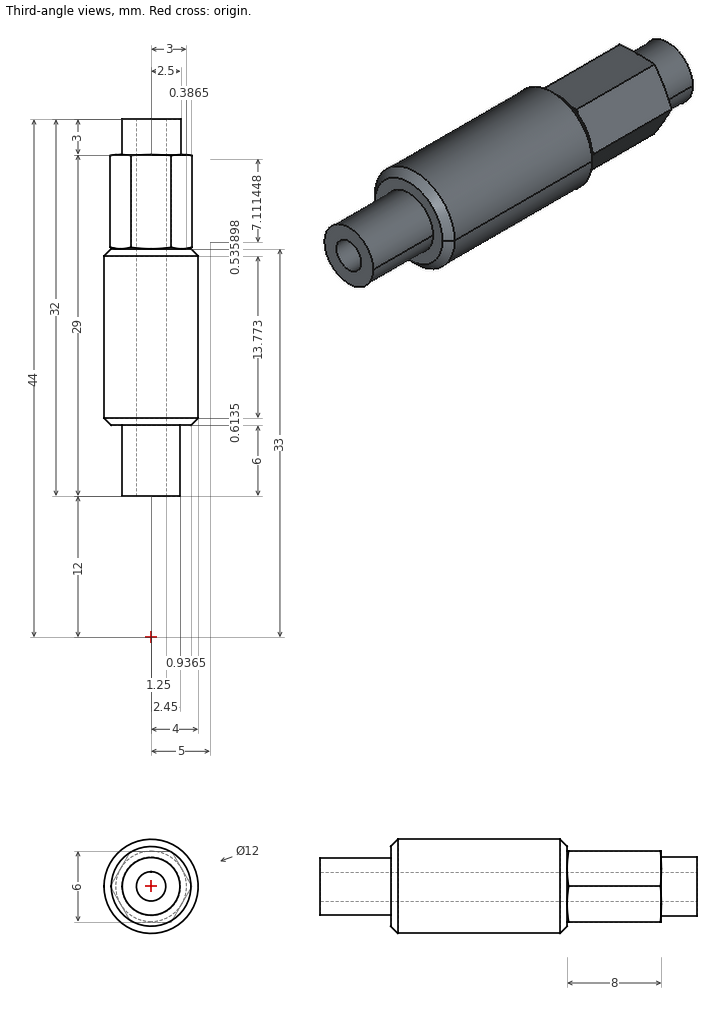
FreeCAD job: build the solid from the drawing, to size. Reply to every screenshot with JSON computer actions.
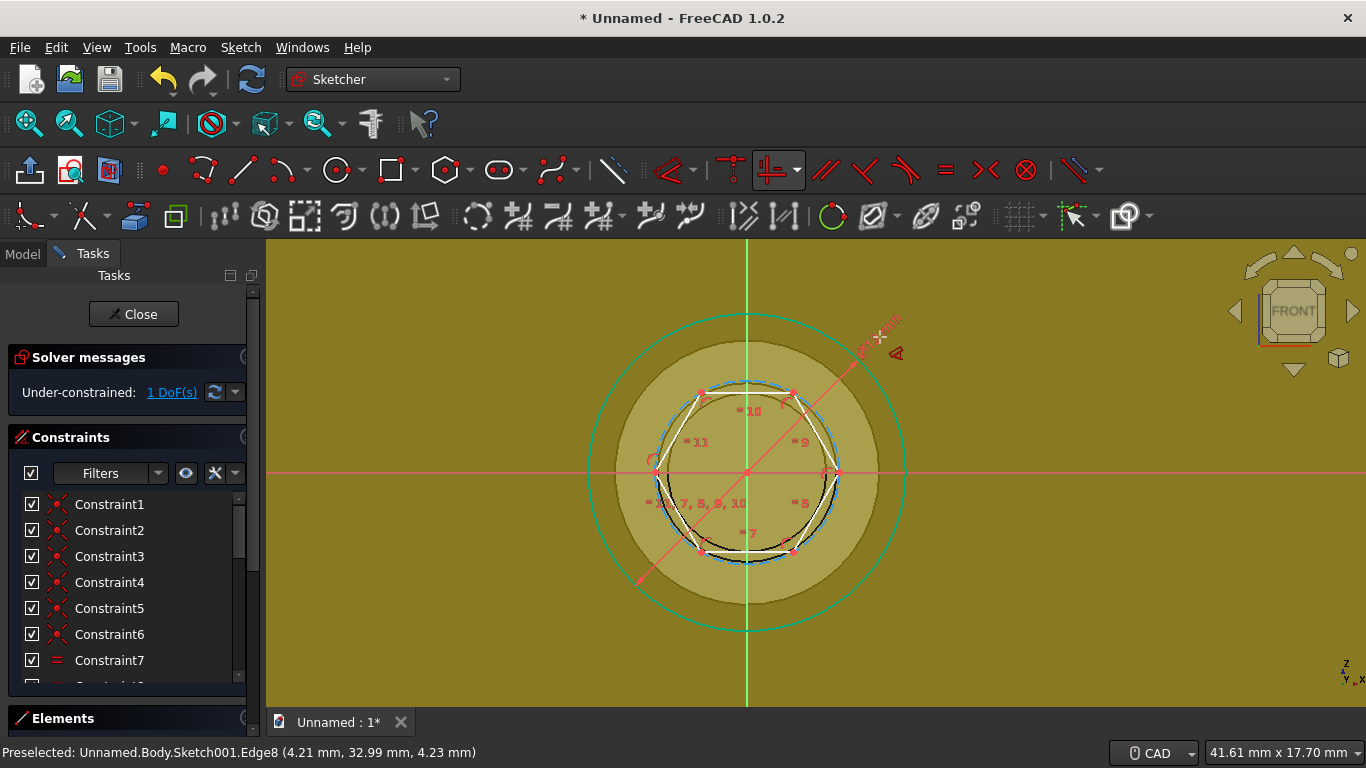
{"action": "left_click", "coordinate": [701, 552]}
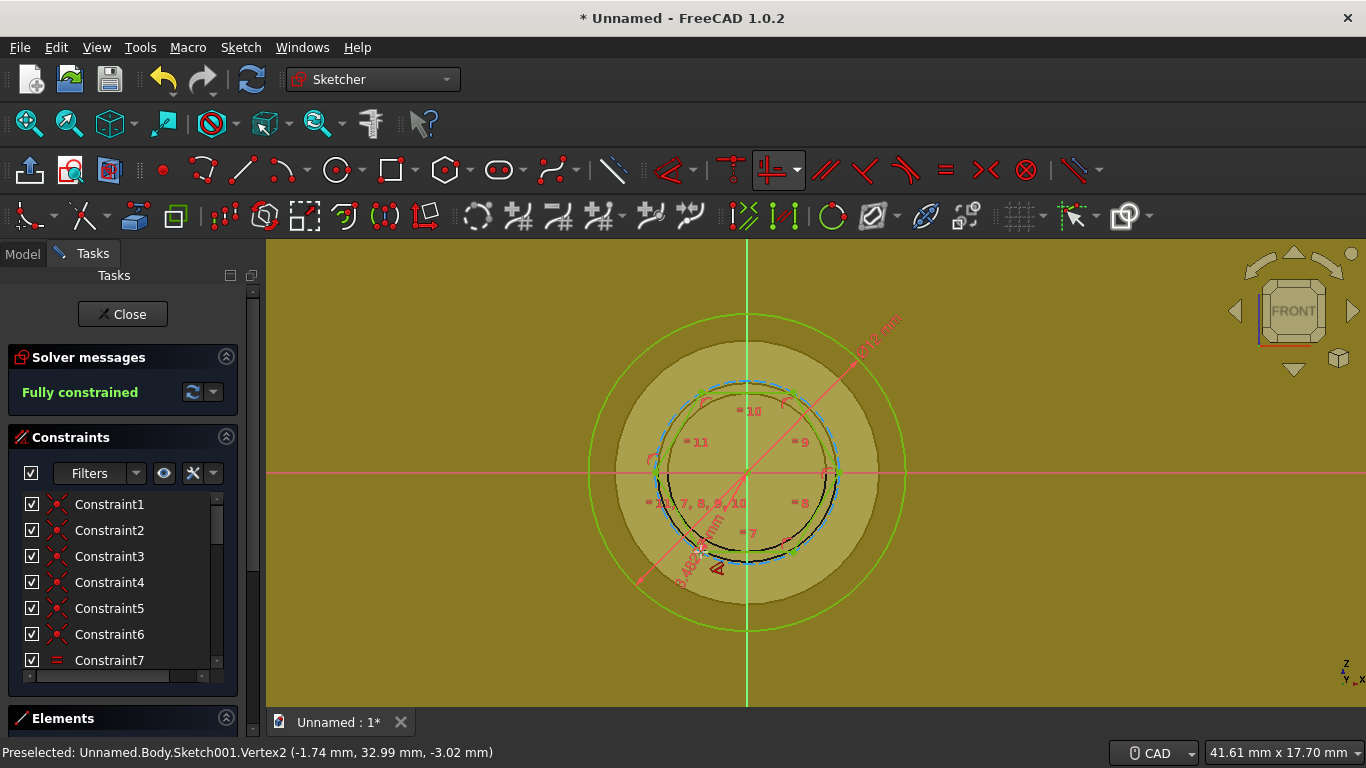
{"action": "left_click", "coordinate": [793, 393]}
{"action": "left_click", "coordinate": [851, 436]}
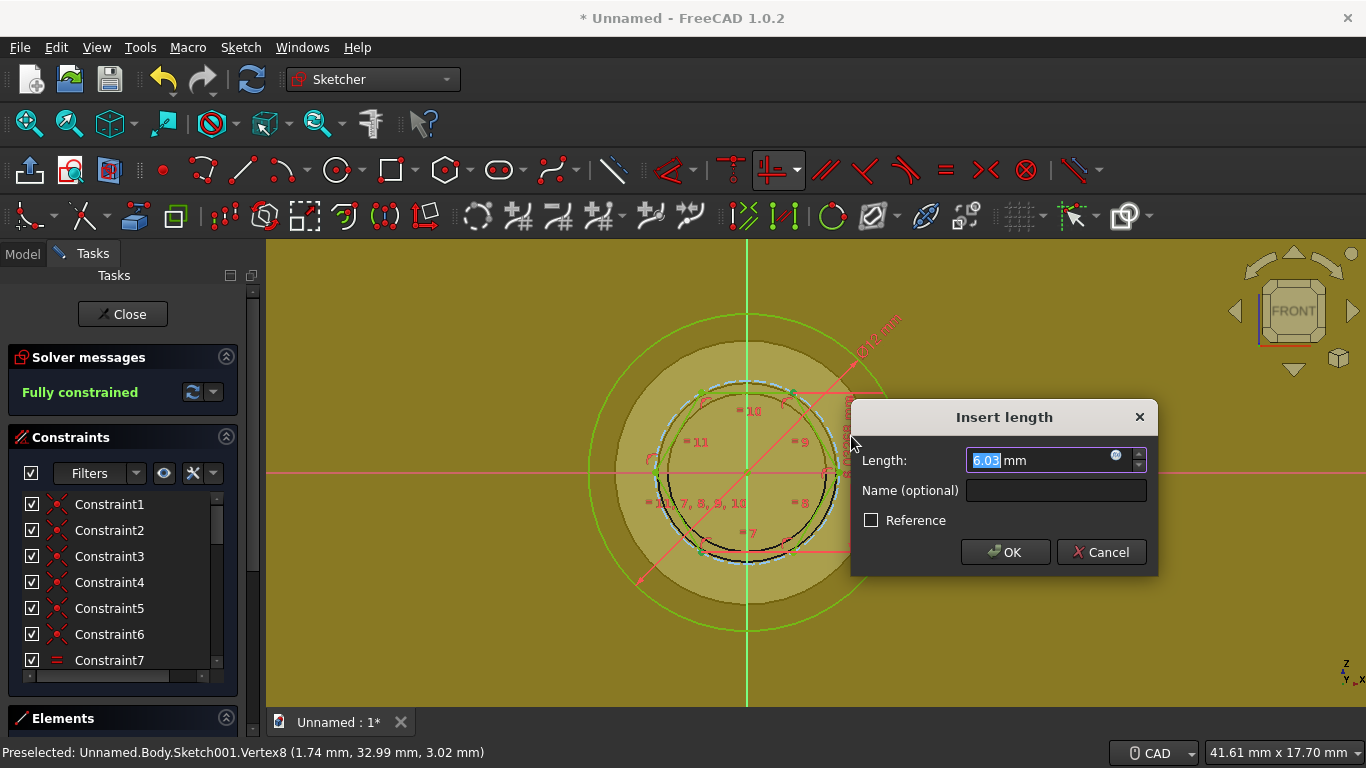
{"action": "type", "text": "6"}
{"action": "key", "text": "Return"}
{"action": "key", "text": "Escape"}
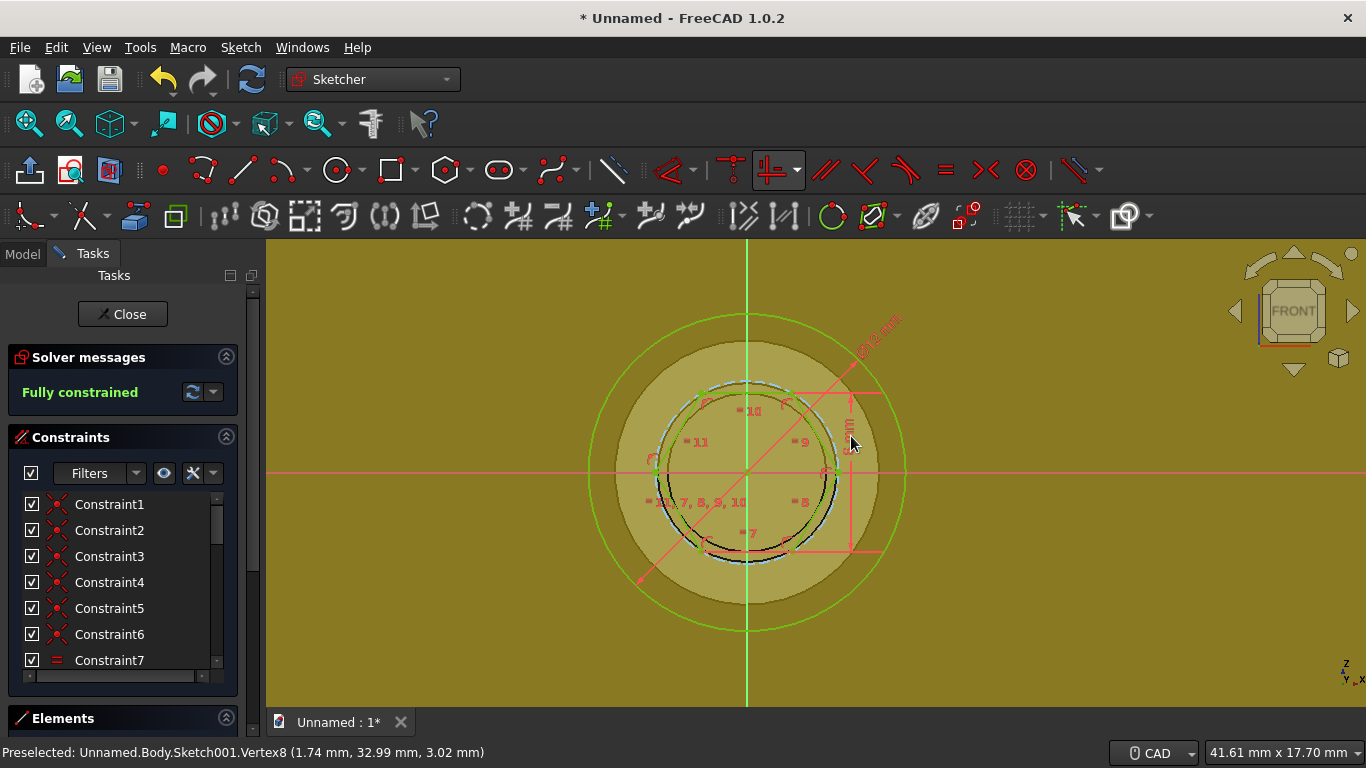
{"action": "left_click", "coordinate": [123, 314]}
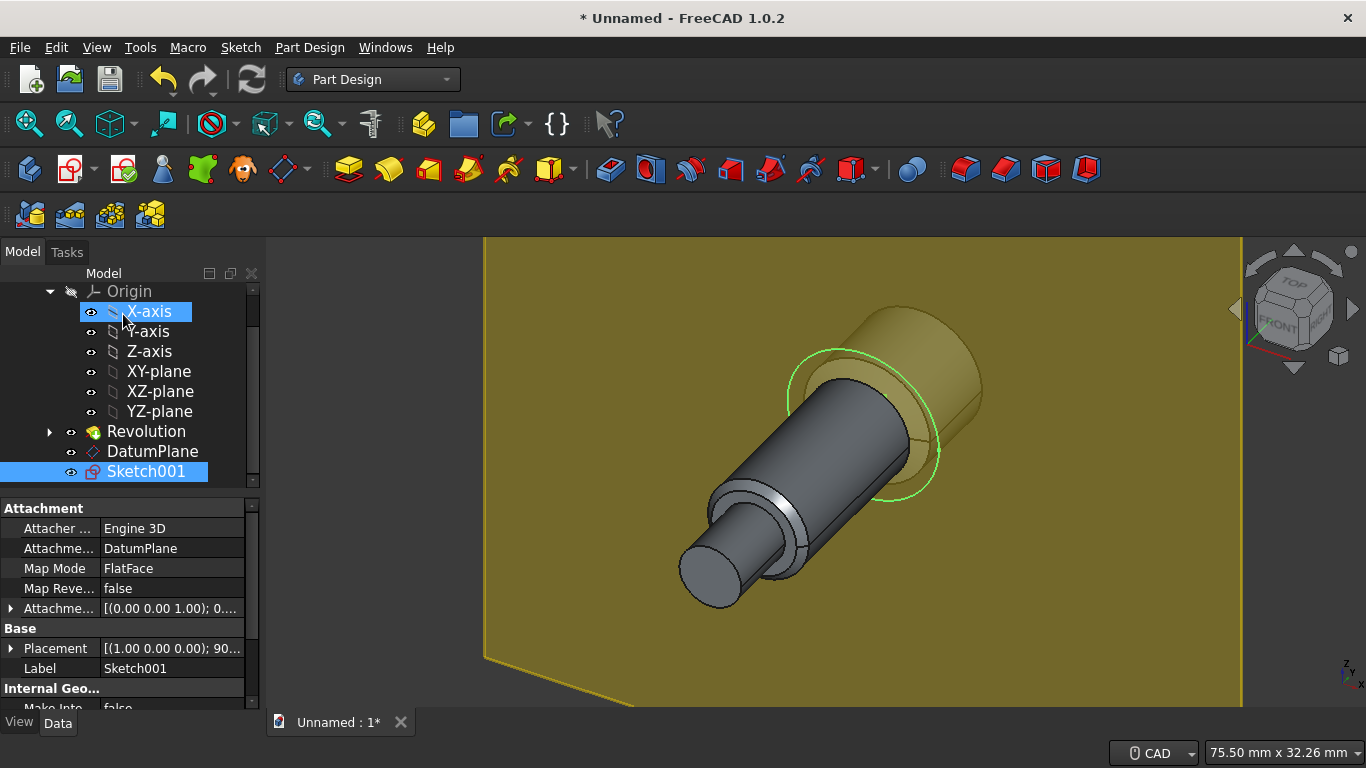
{"action": "left_click", "coordinate": [612, 170]}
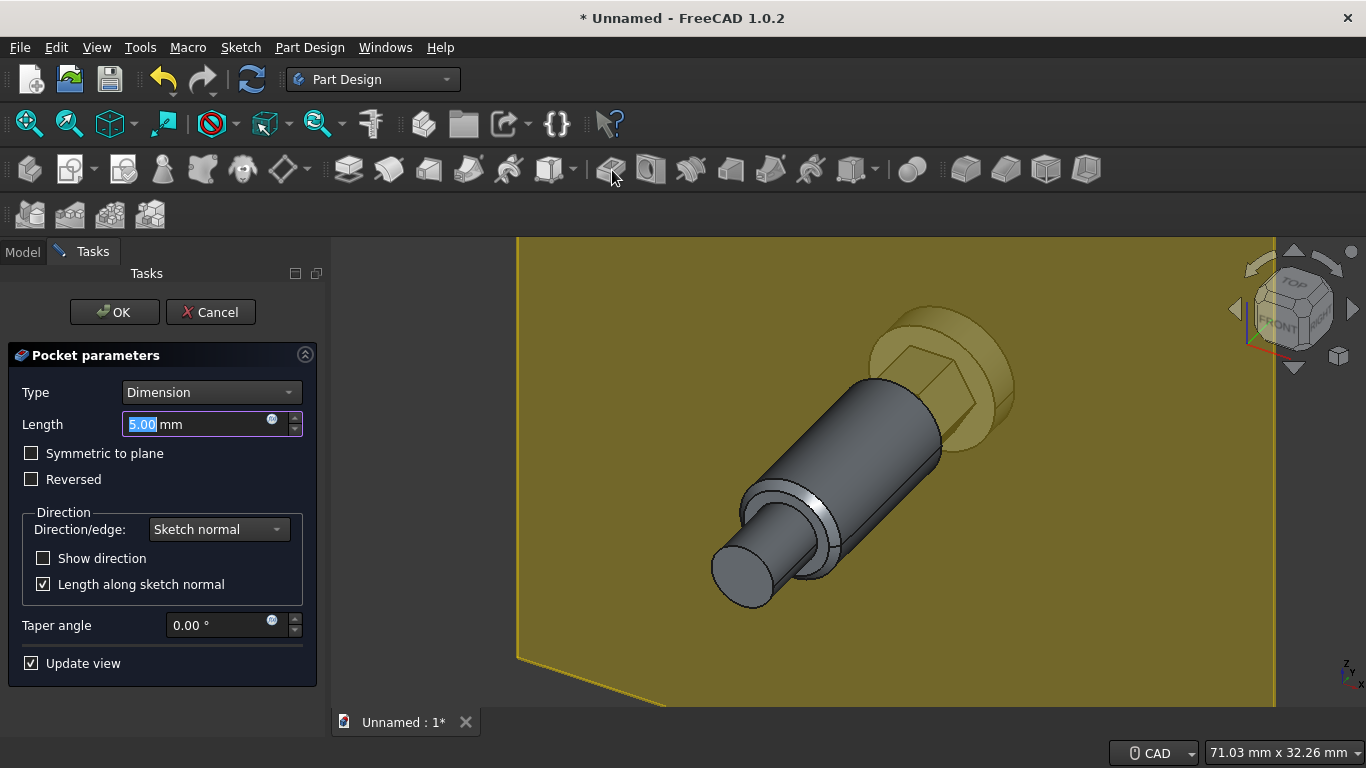
{"action": "type", "text": "8"}
{"action": "key", "text": "Tab"}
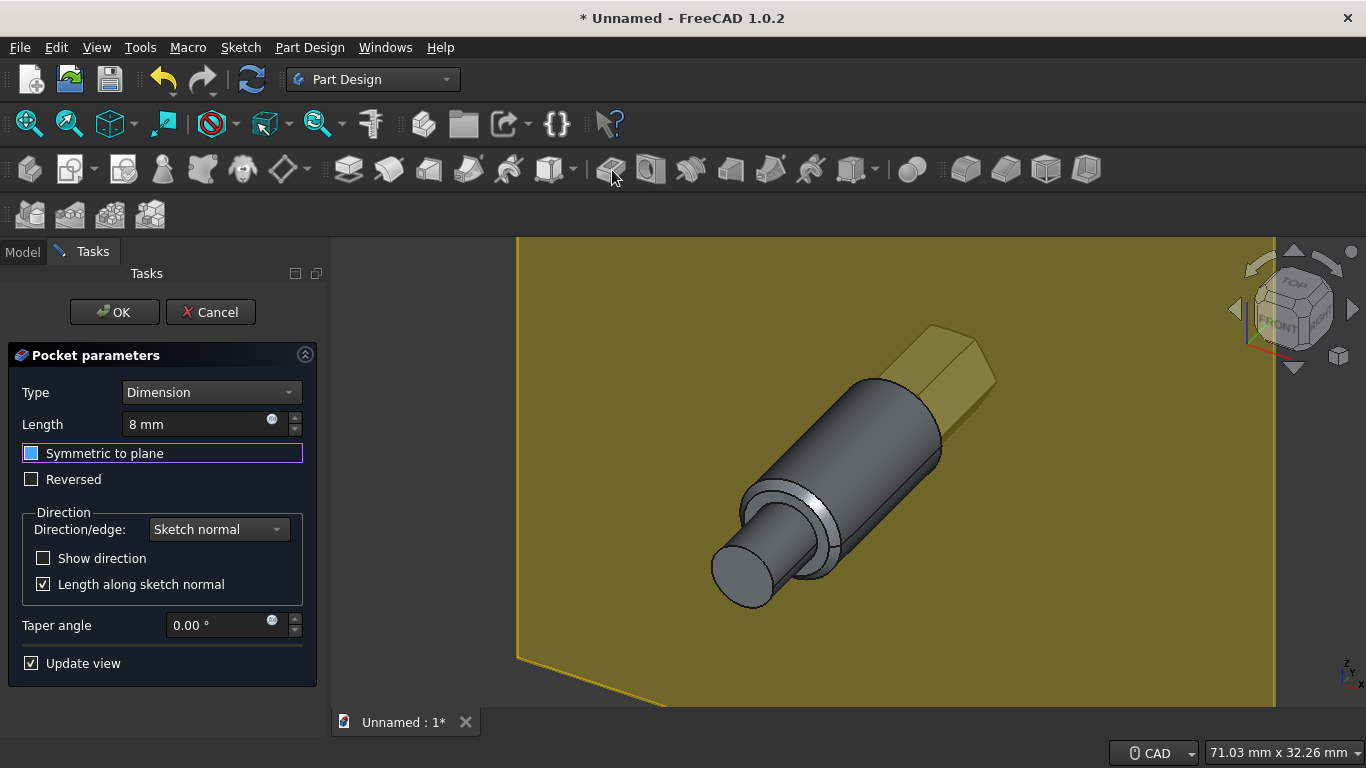
{"action": "left_click", "coordinate": [115, 312]}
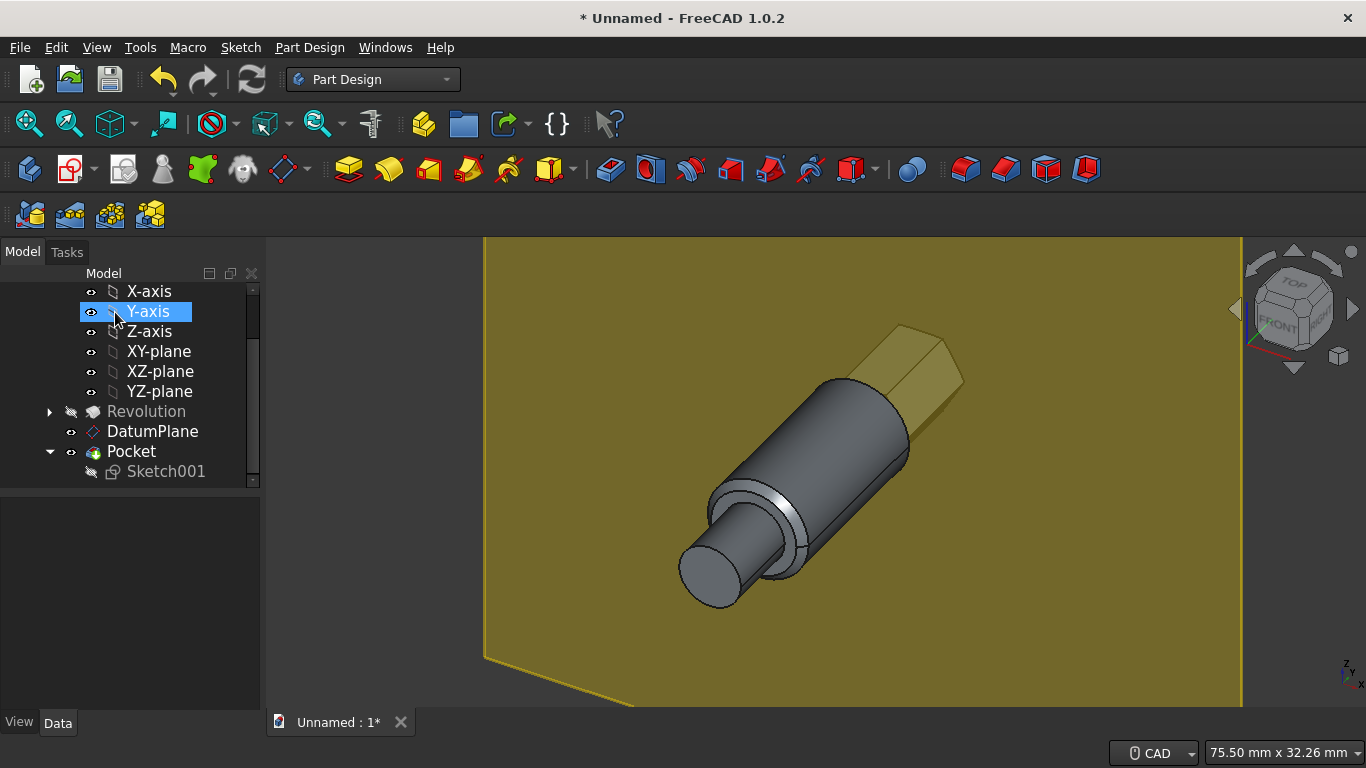
{"action": "left_click", "coordinate": [116, 432]}
{"action": "key", "text": "space"}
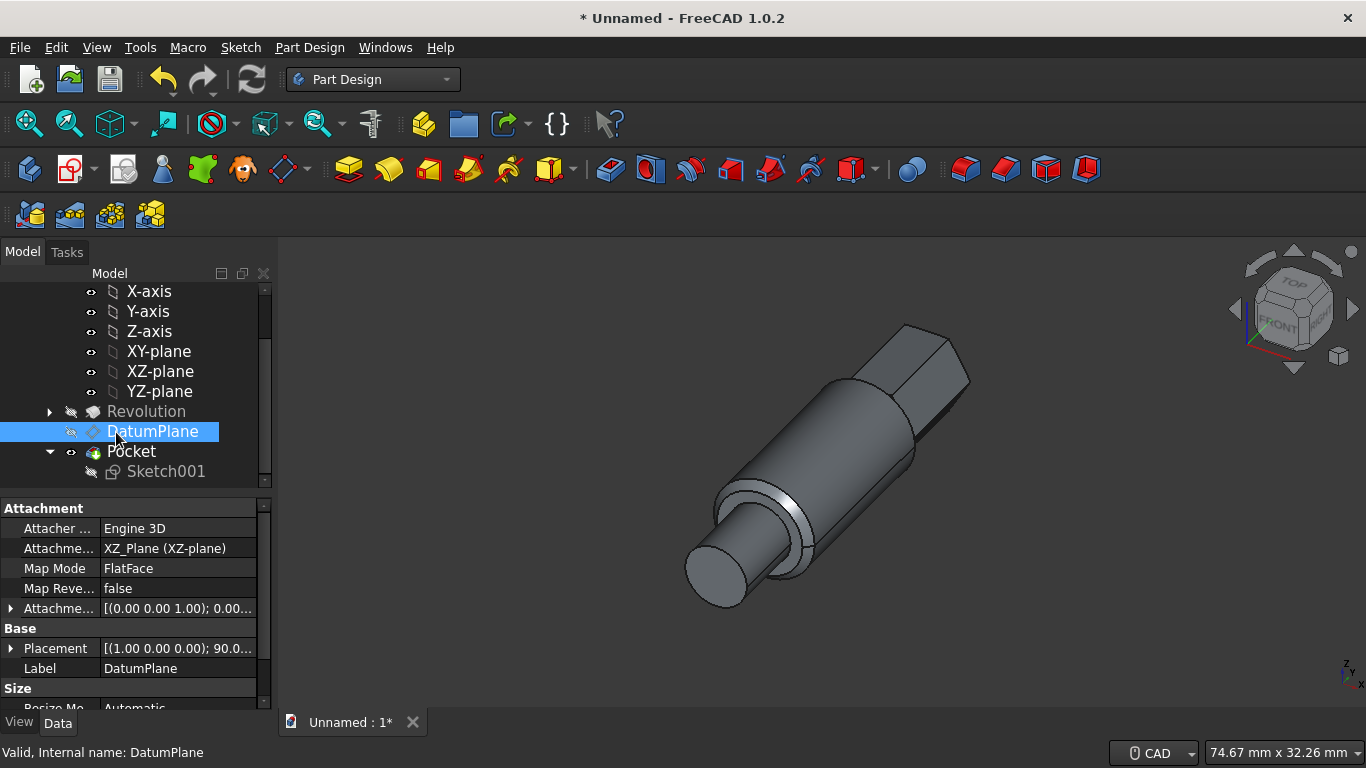
{"action": "left_click", "coordinate": [318, 667]}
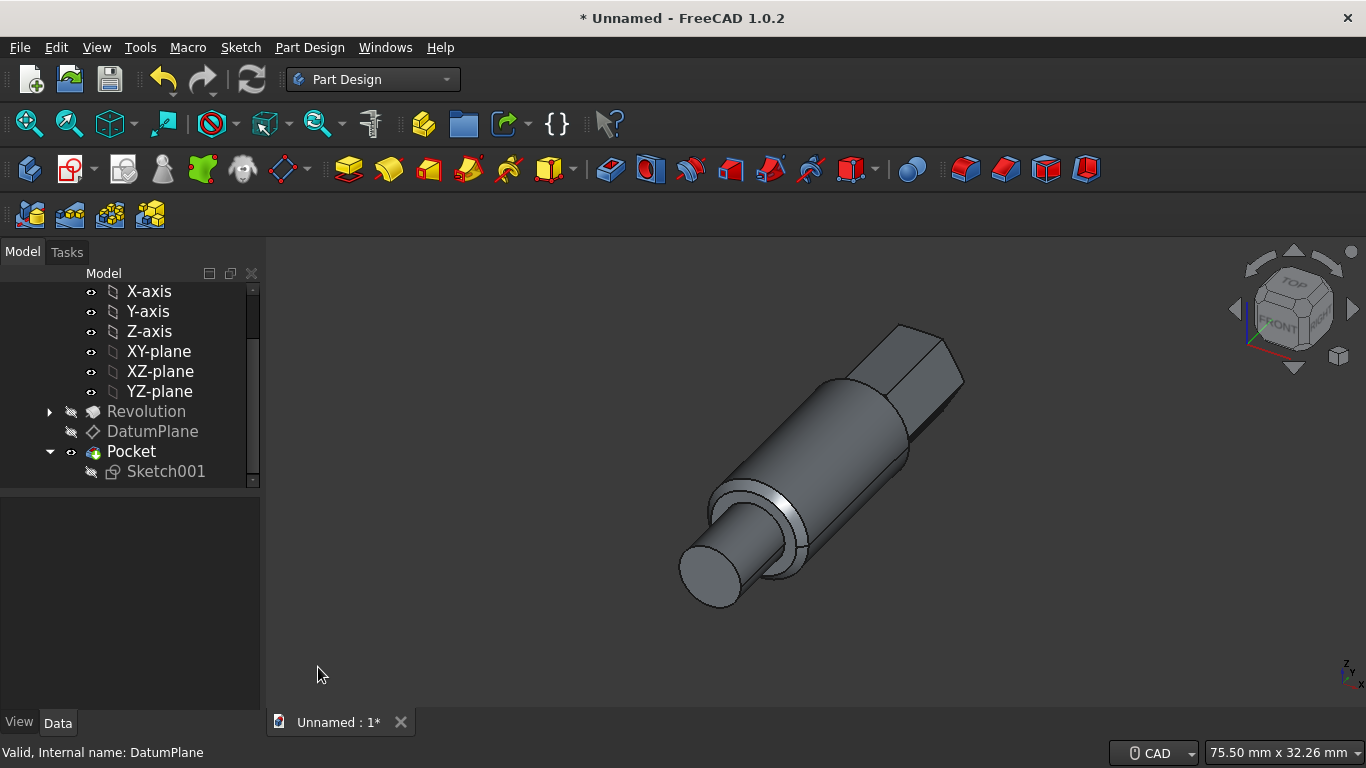
{"action": "left_click", "coordinate": [70, 170]}